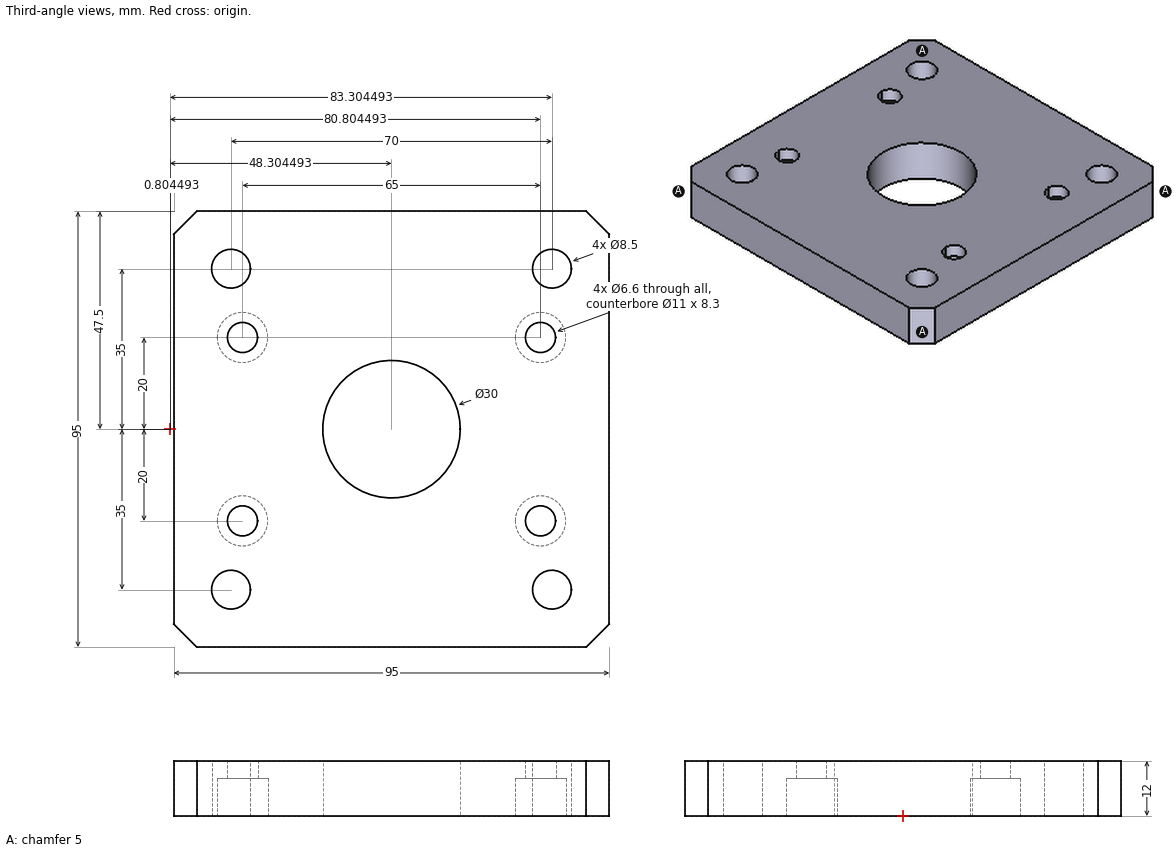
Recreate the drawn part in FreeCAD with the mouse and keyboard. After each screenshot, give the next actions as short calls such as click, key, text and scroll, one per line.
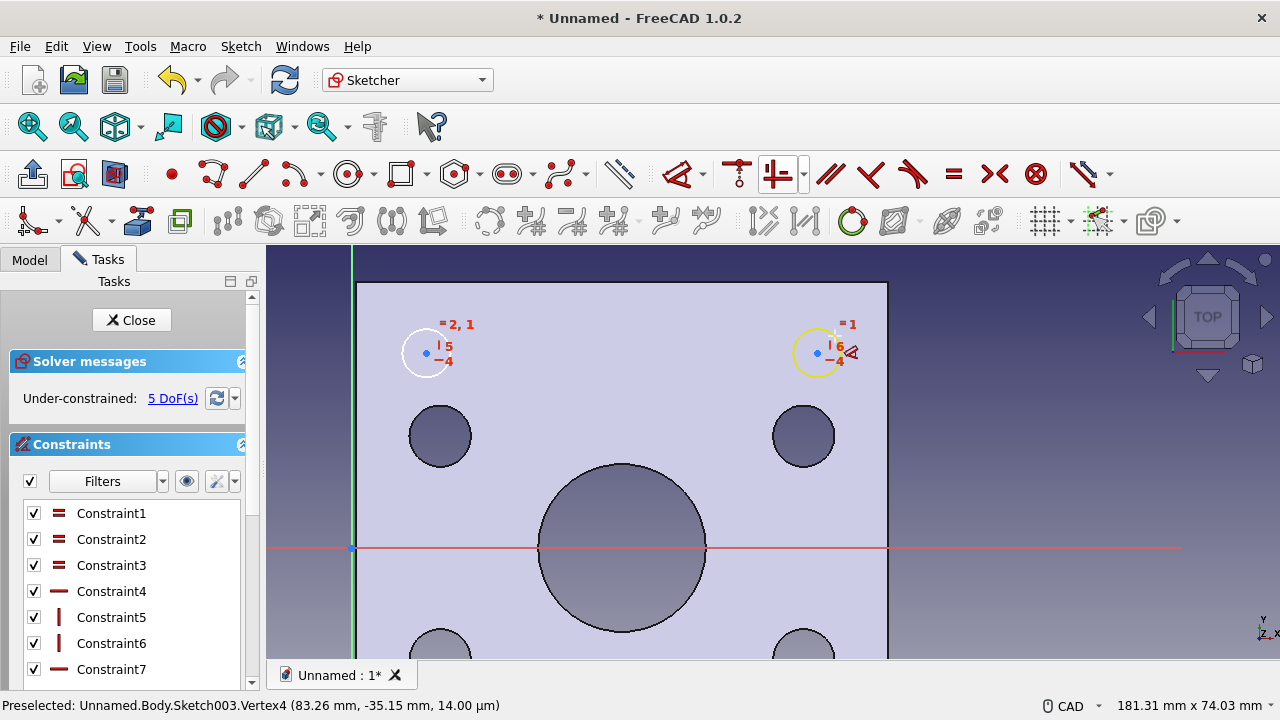
click(834, 336)
click(856, 313)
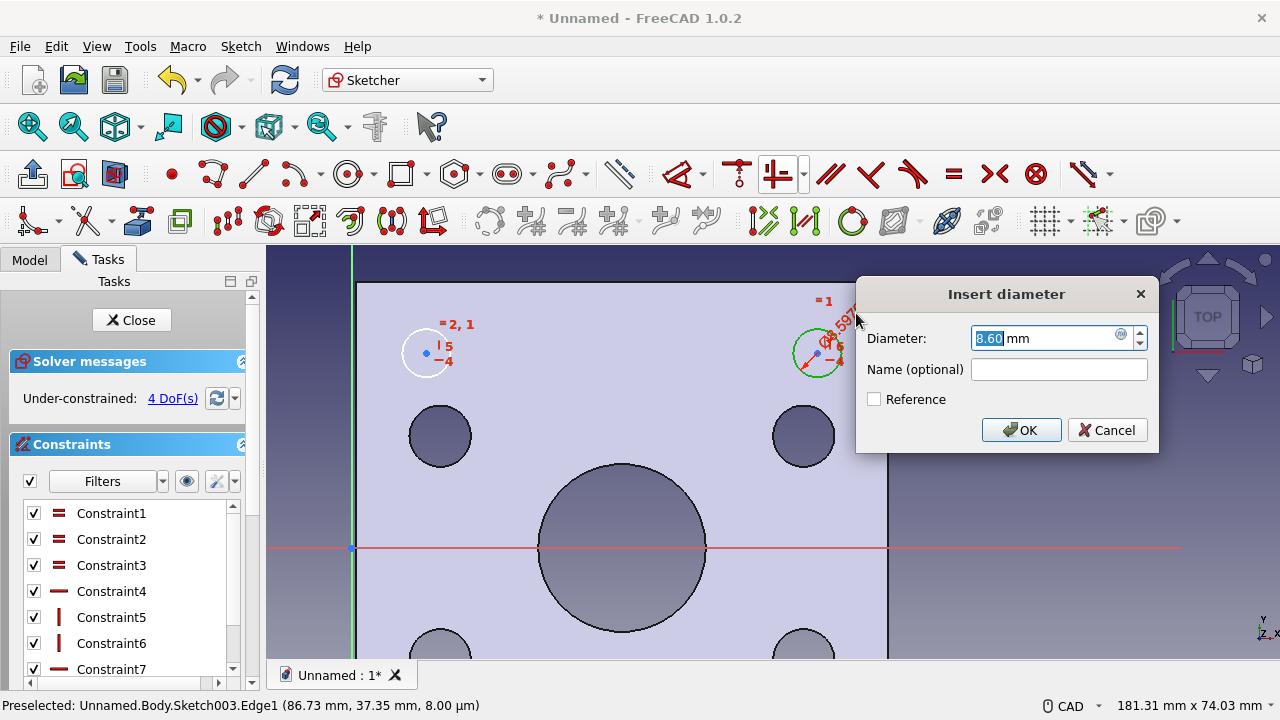
text(8.5)
key(Return)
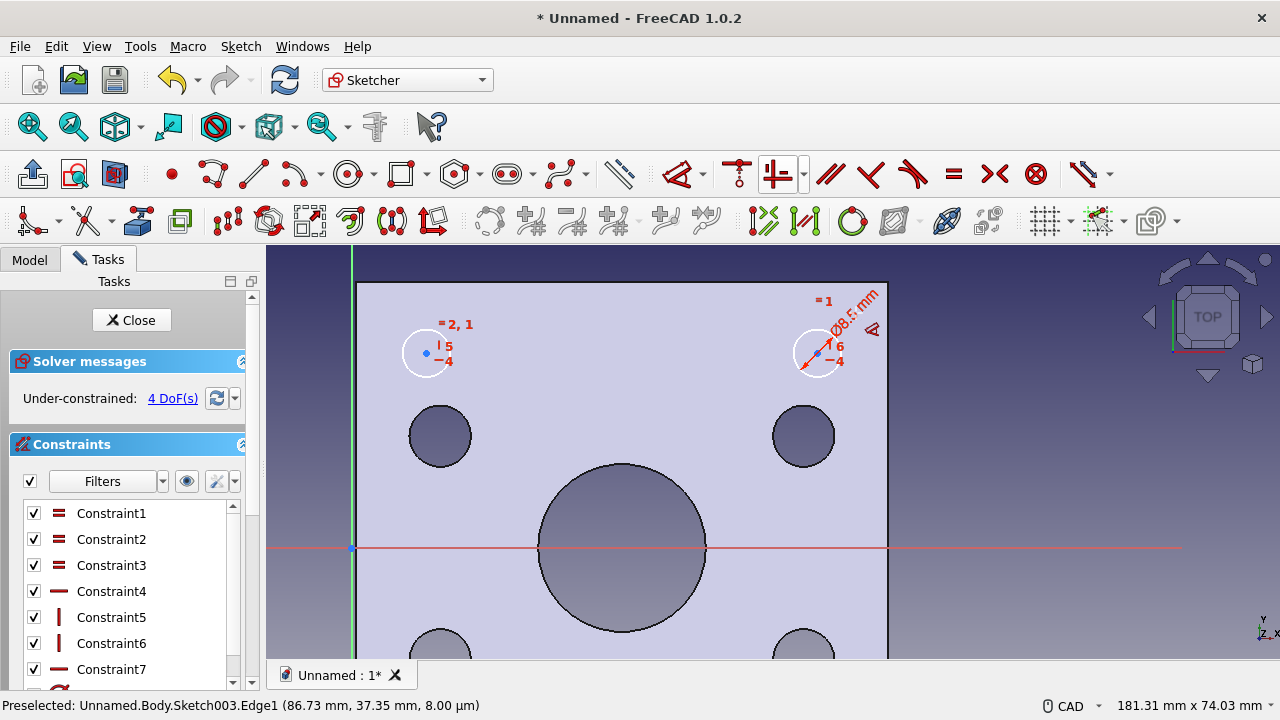
click(817, 353)
click(318, 451)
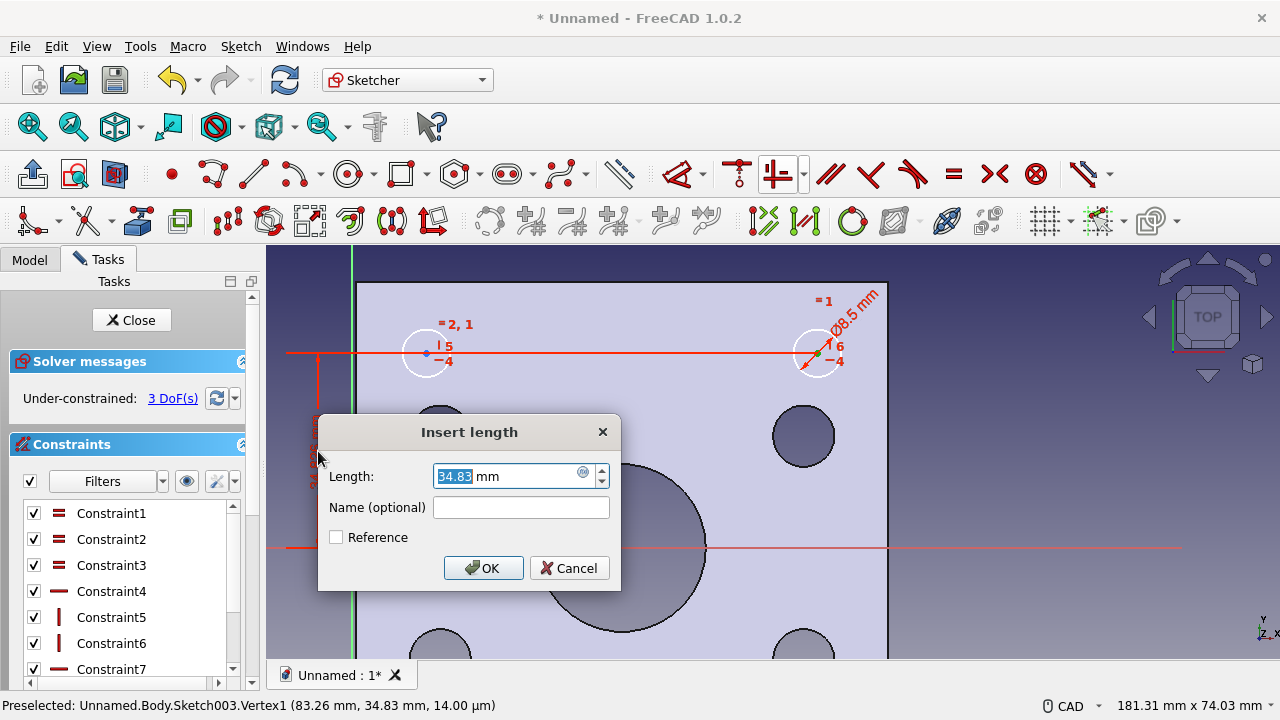
text(35)
key(Return)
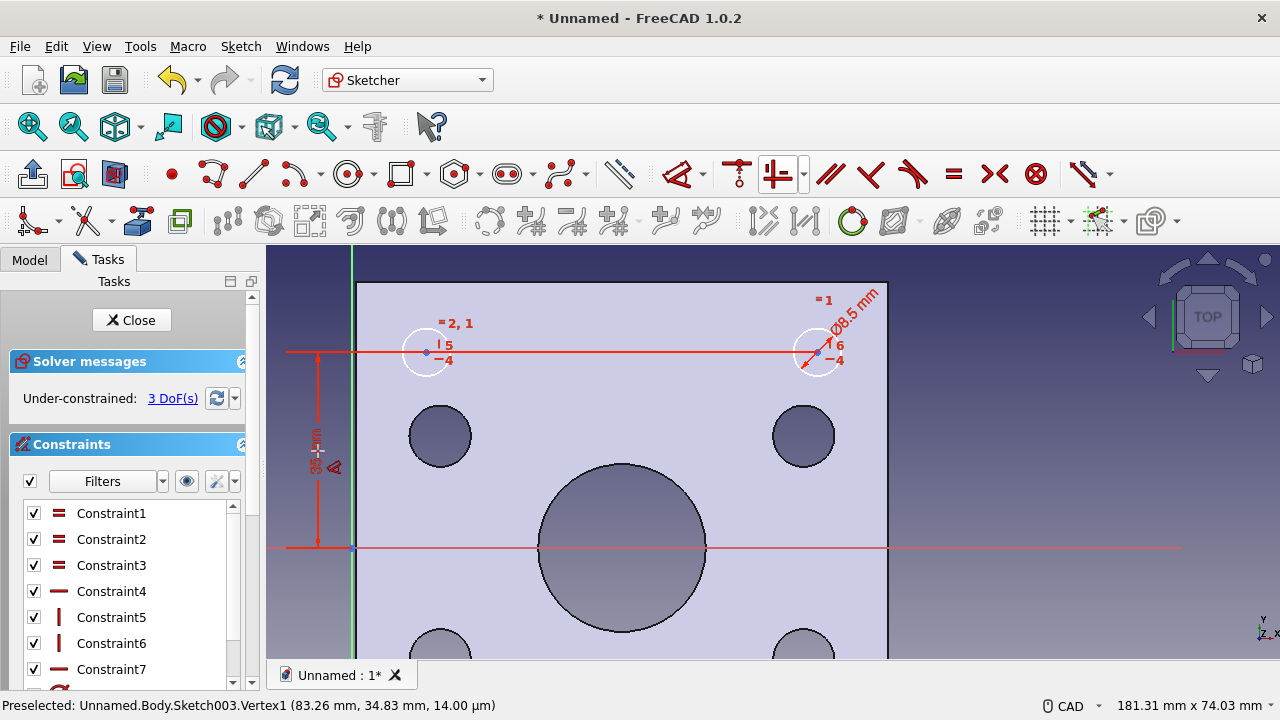
scroll(836, 335, down, 3)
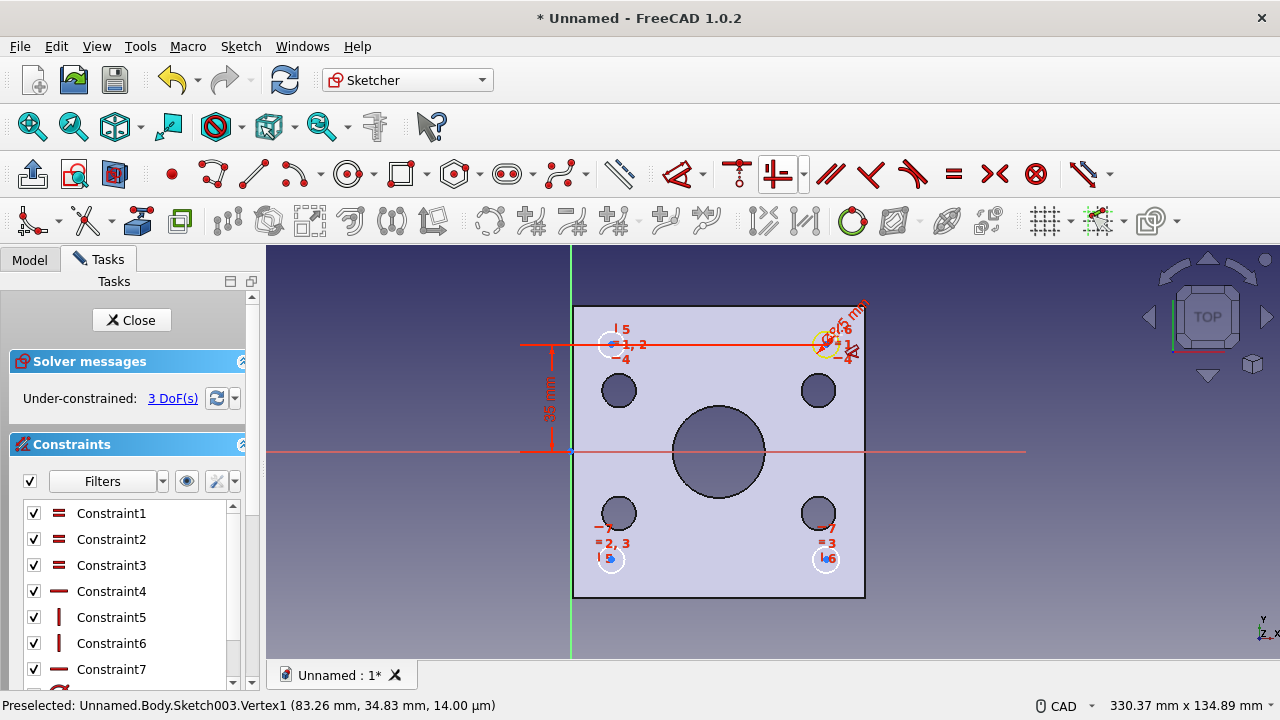
click(611, 560)
click(537, 506)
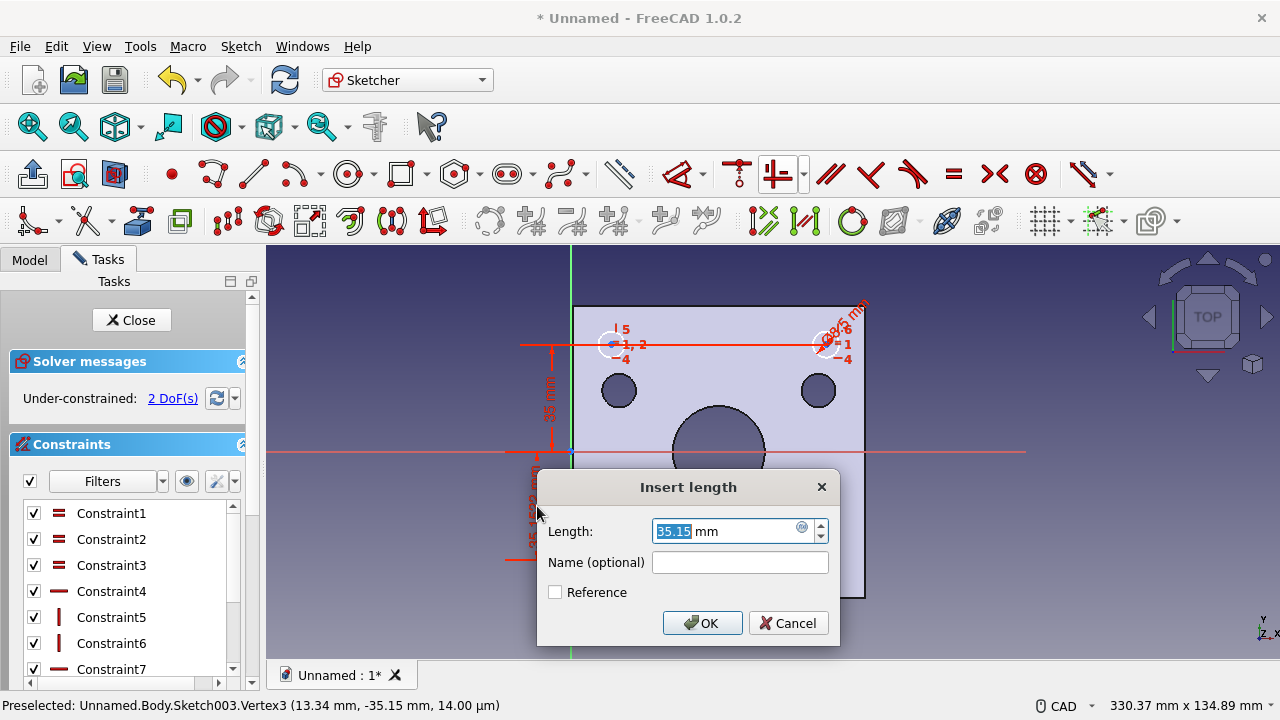
text(35)
key(Return)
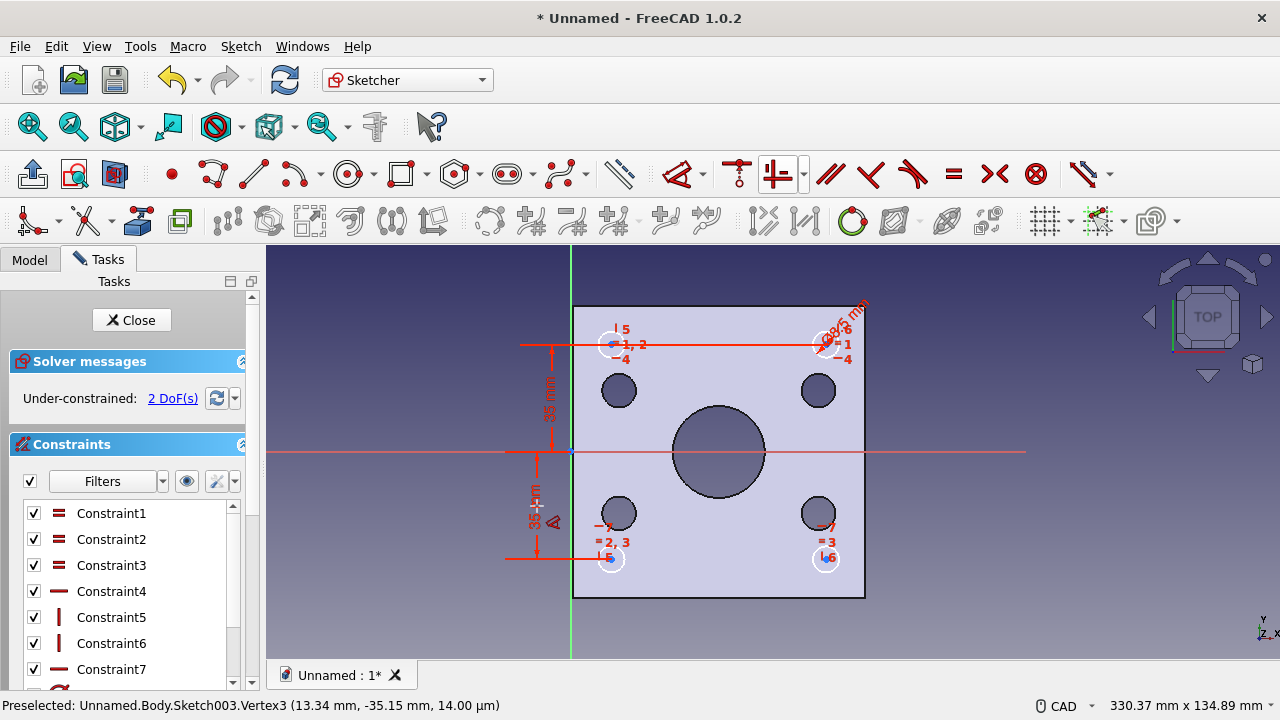
click(826, 345)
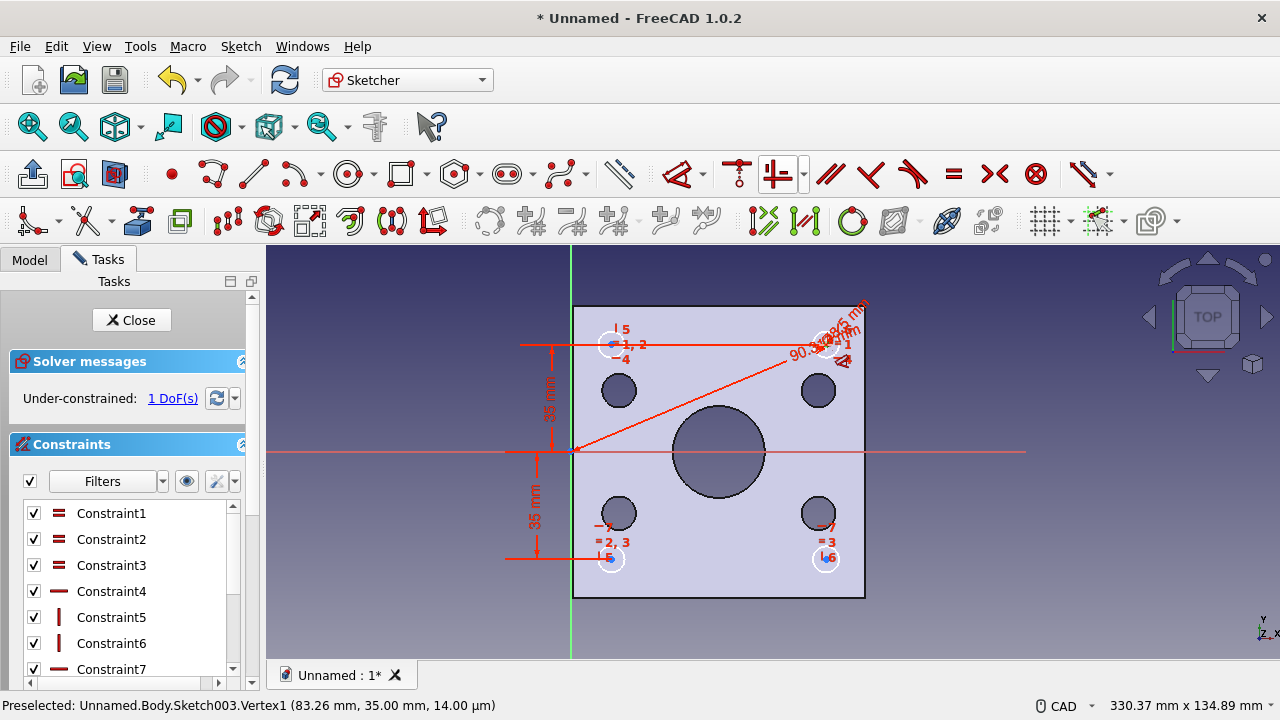
click(611, 345)
click(719, 311)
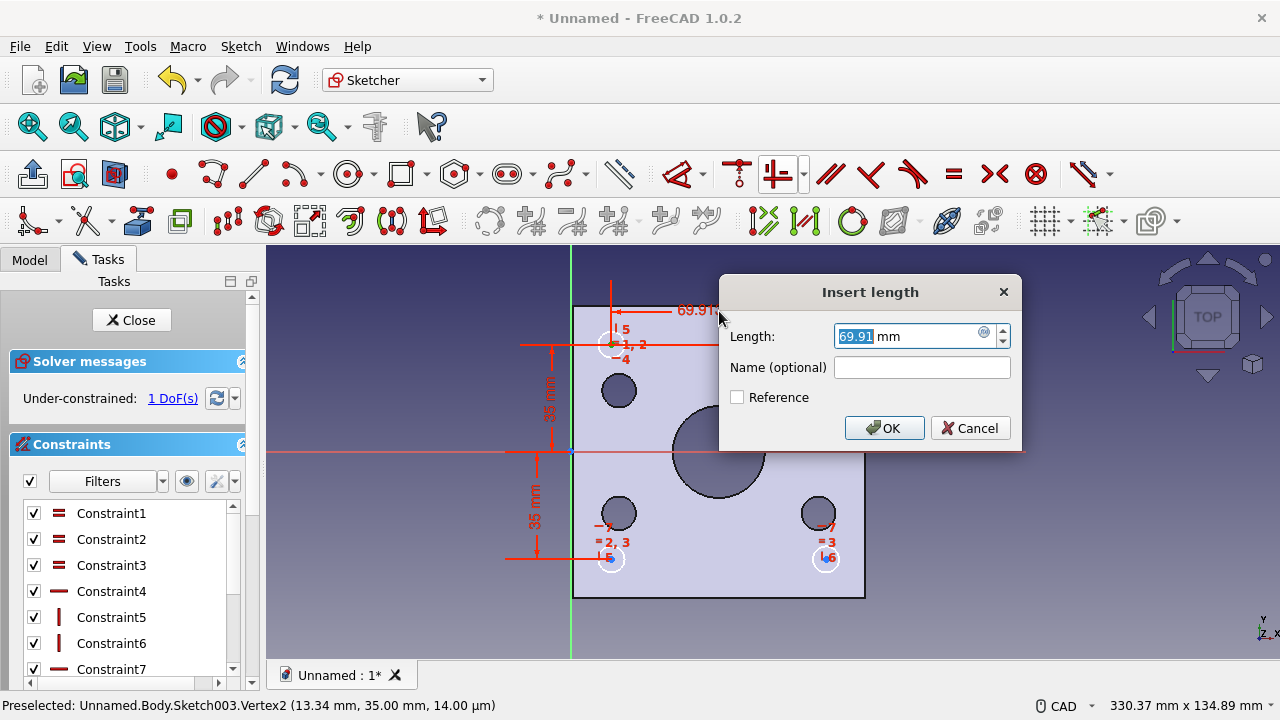
text(70)
key(Return)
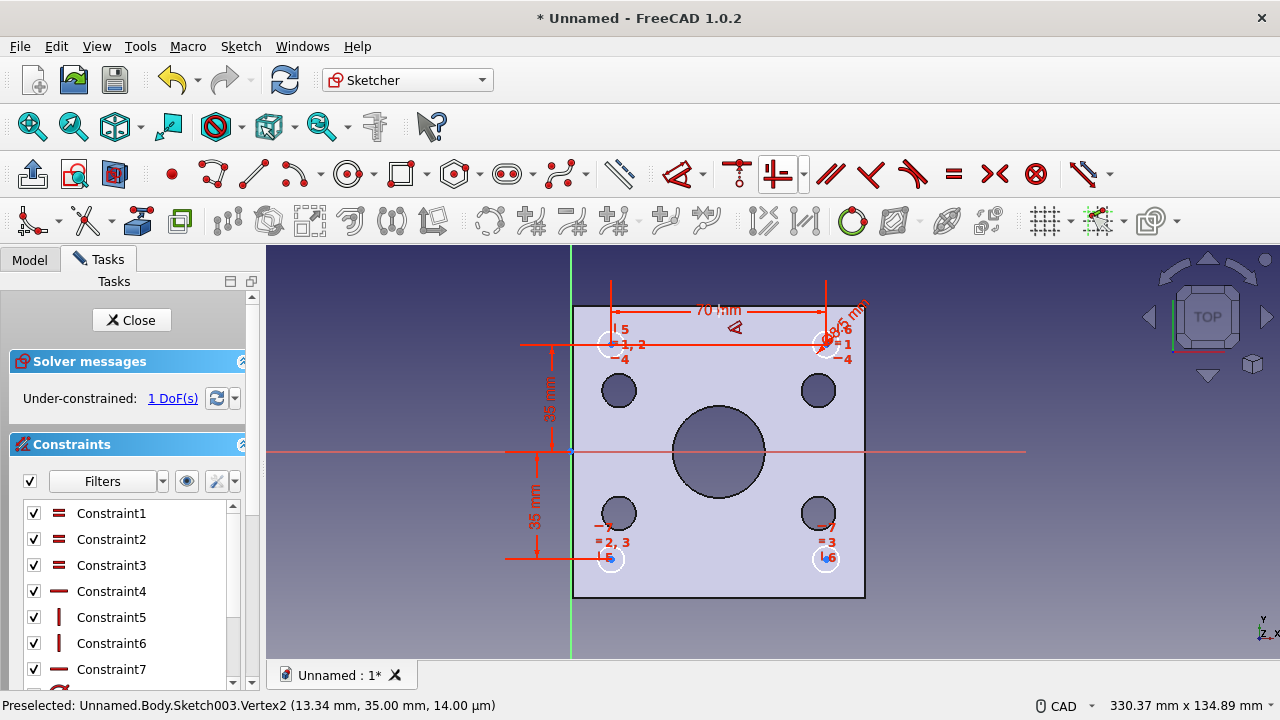
click(826, 345)
click(640, 311)